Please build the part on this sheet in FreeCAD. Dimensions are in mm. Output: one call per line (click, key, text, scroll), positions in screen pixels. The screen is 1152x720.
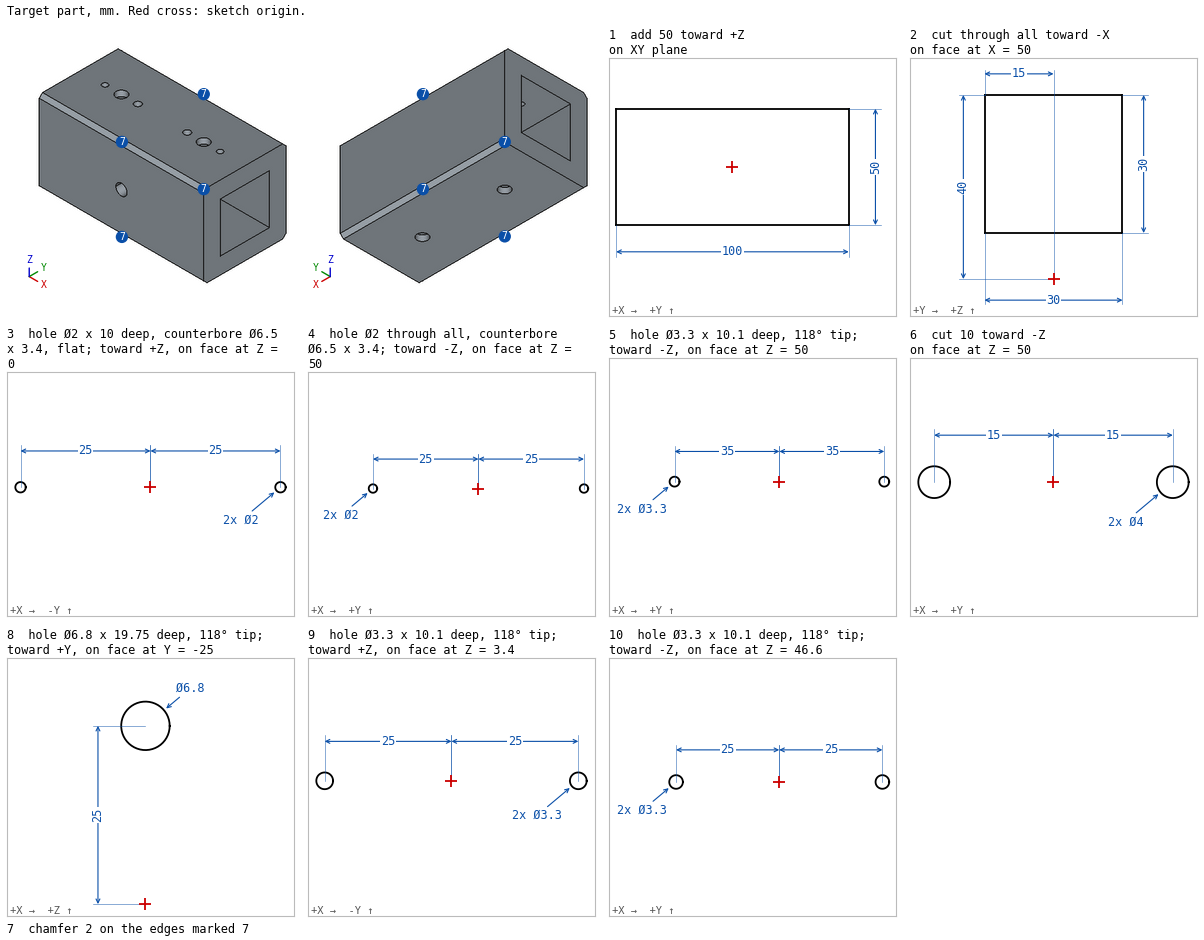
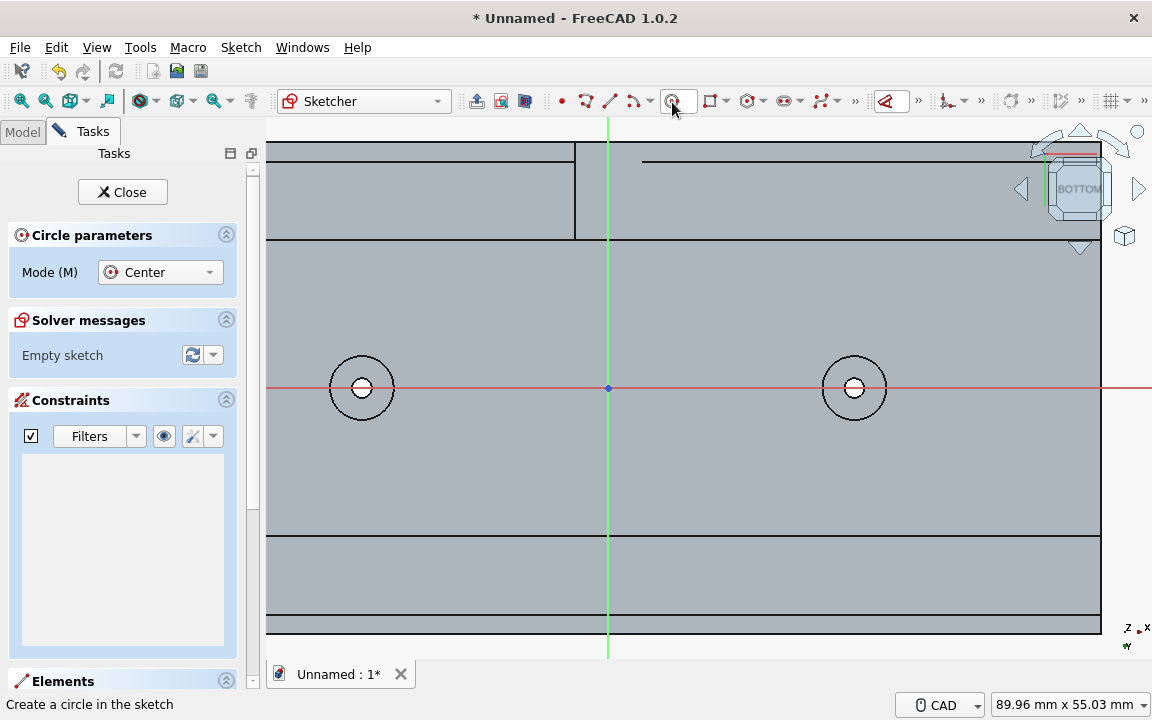
scroll(854, 388, up, 2)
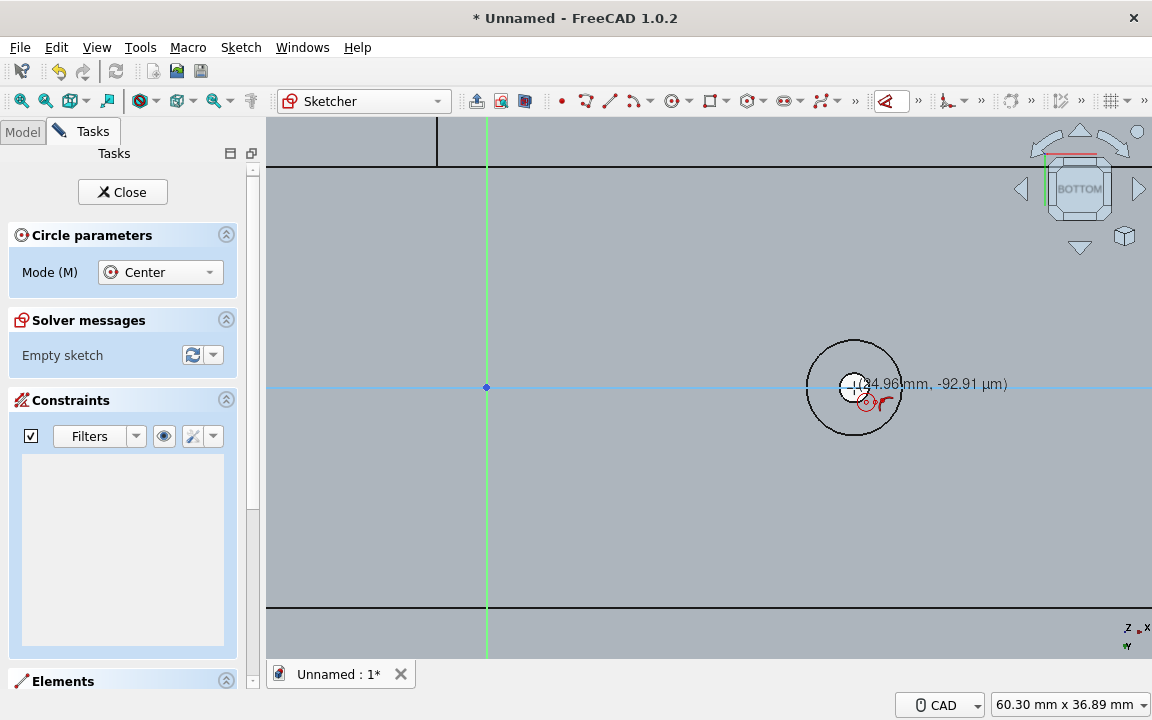
click(854, 388)
move(871, 371)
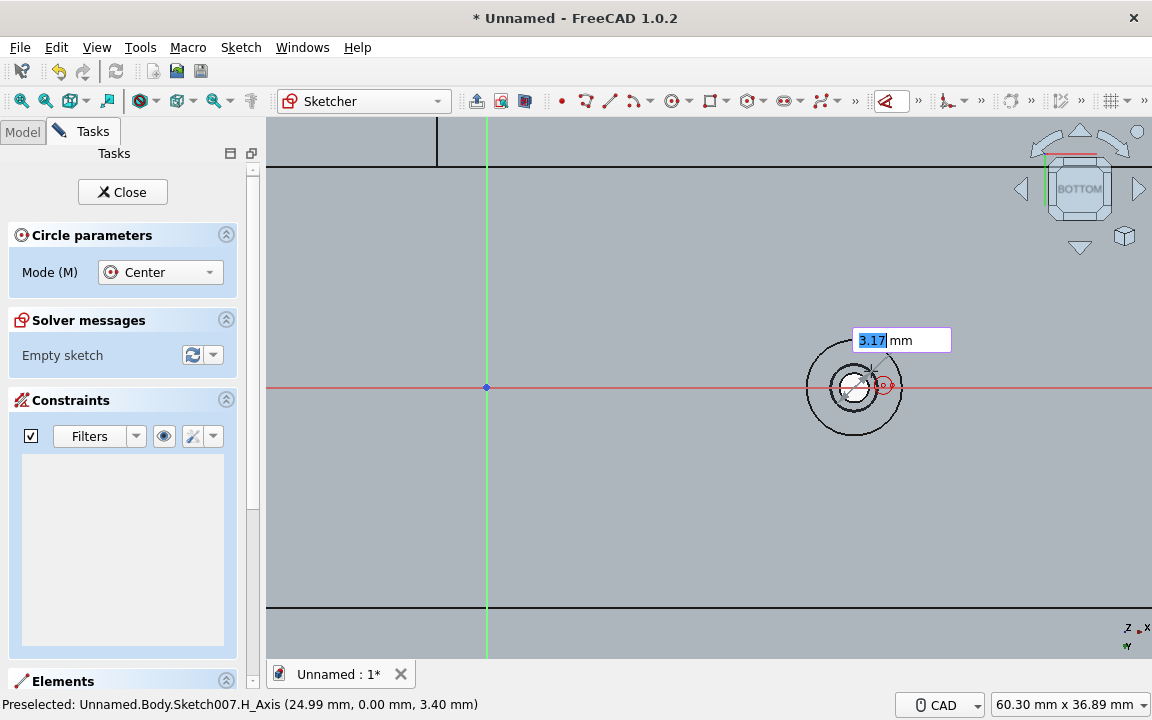
text(3.3)
key(Return)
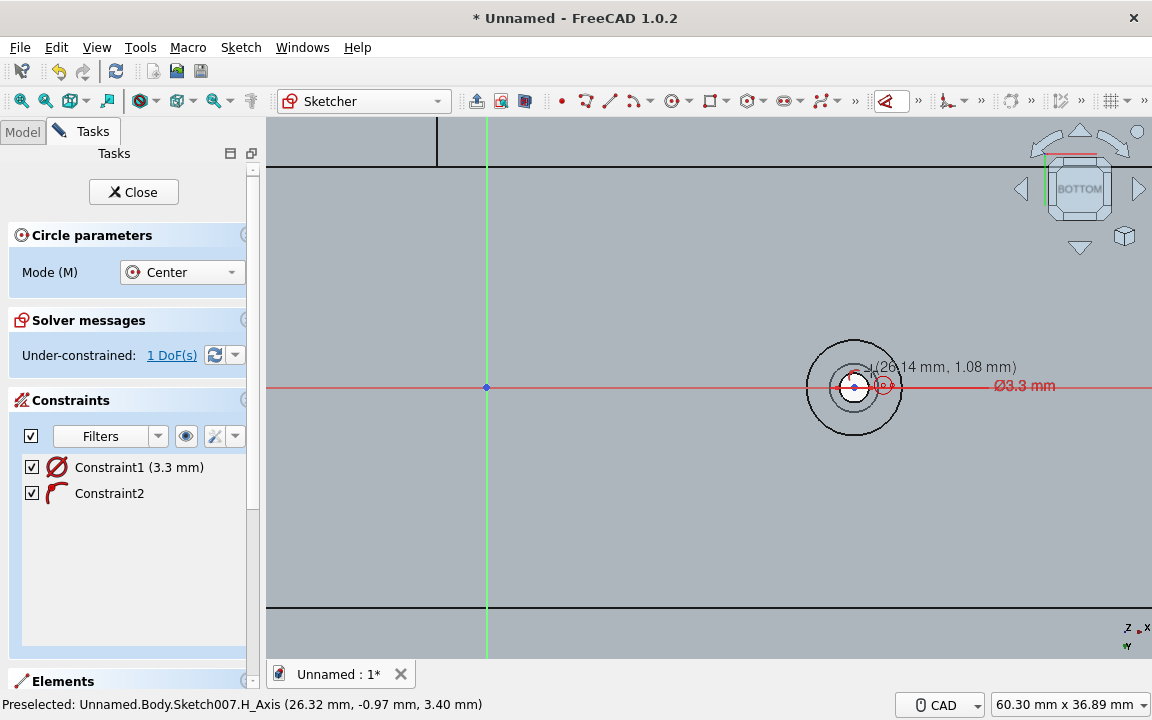
scroll(953, 388, down, 2)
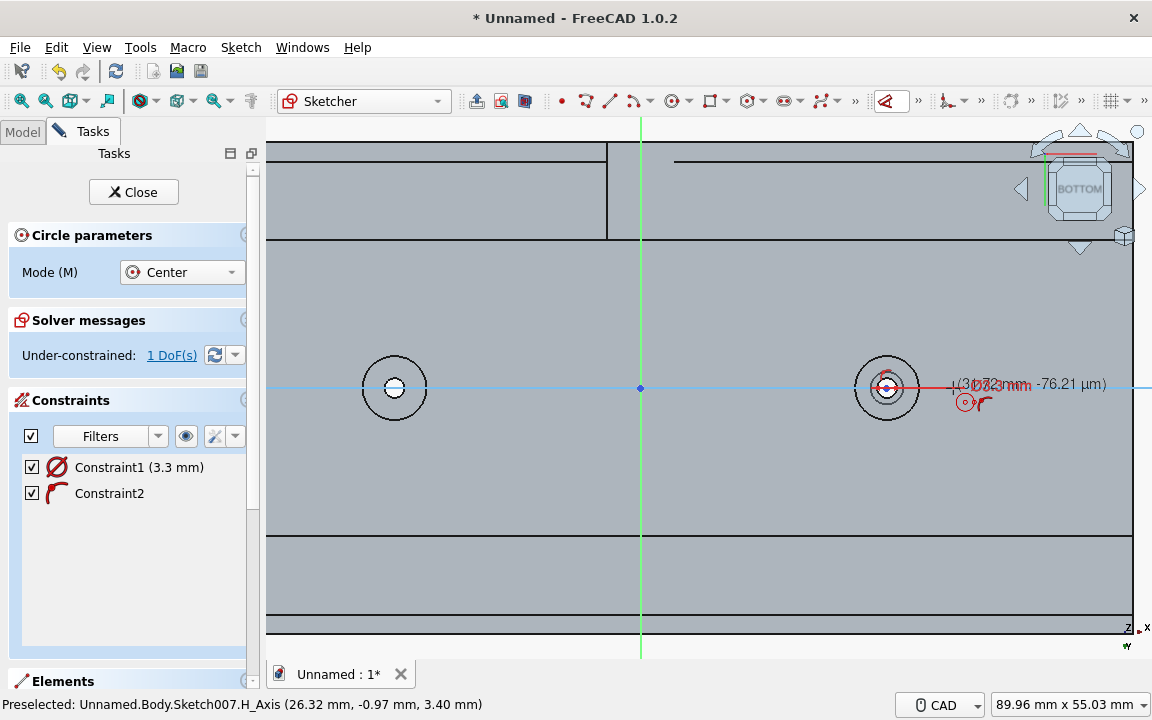
scroll(395, 388, up, 2)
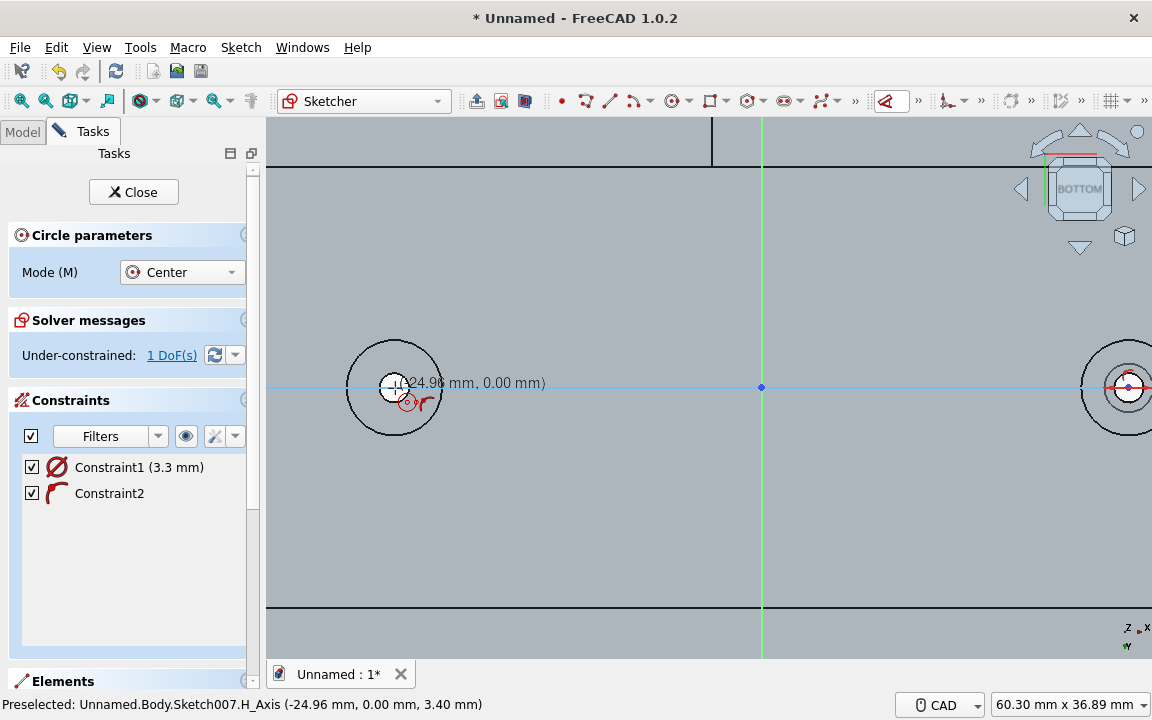
click(394, 388)
move(411, 371)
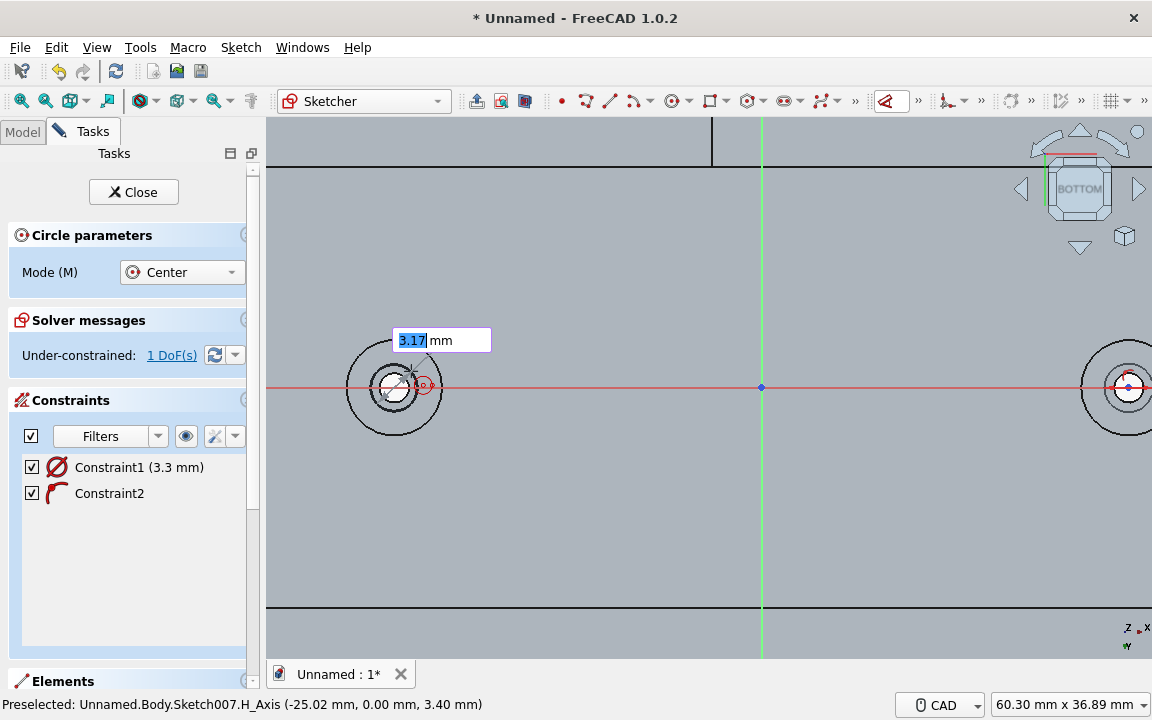
text(3.3)
key(Return)
key(Escape)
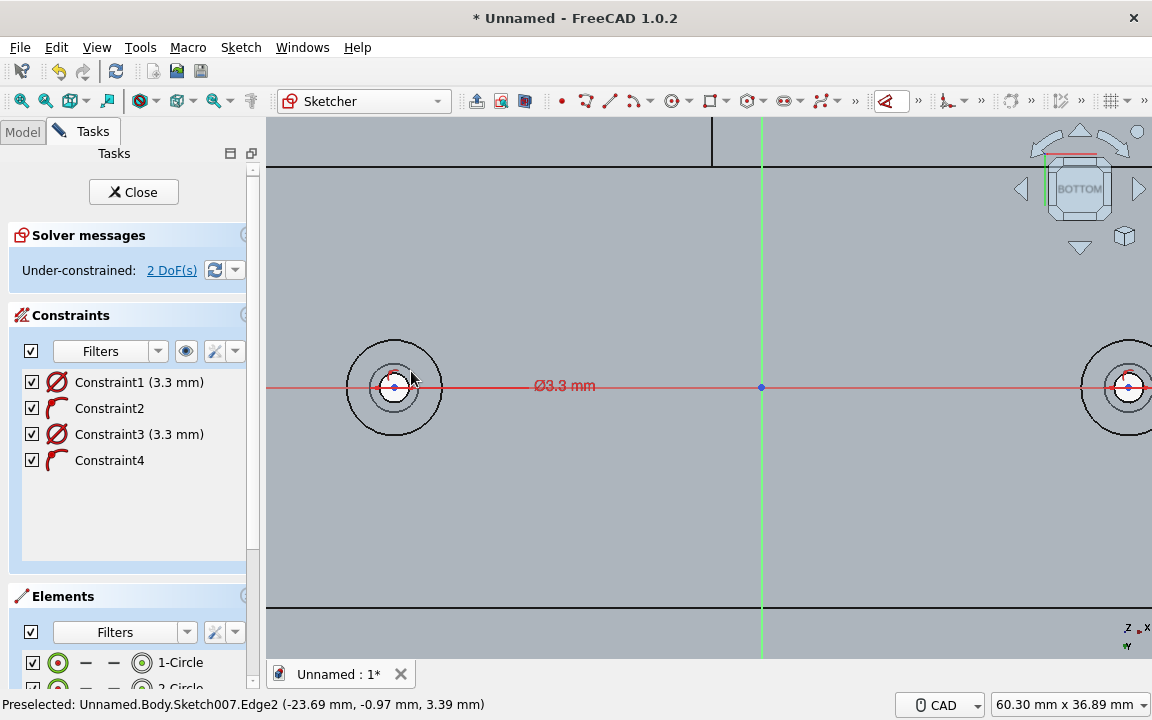
scroll(394, 388, down, 2)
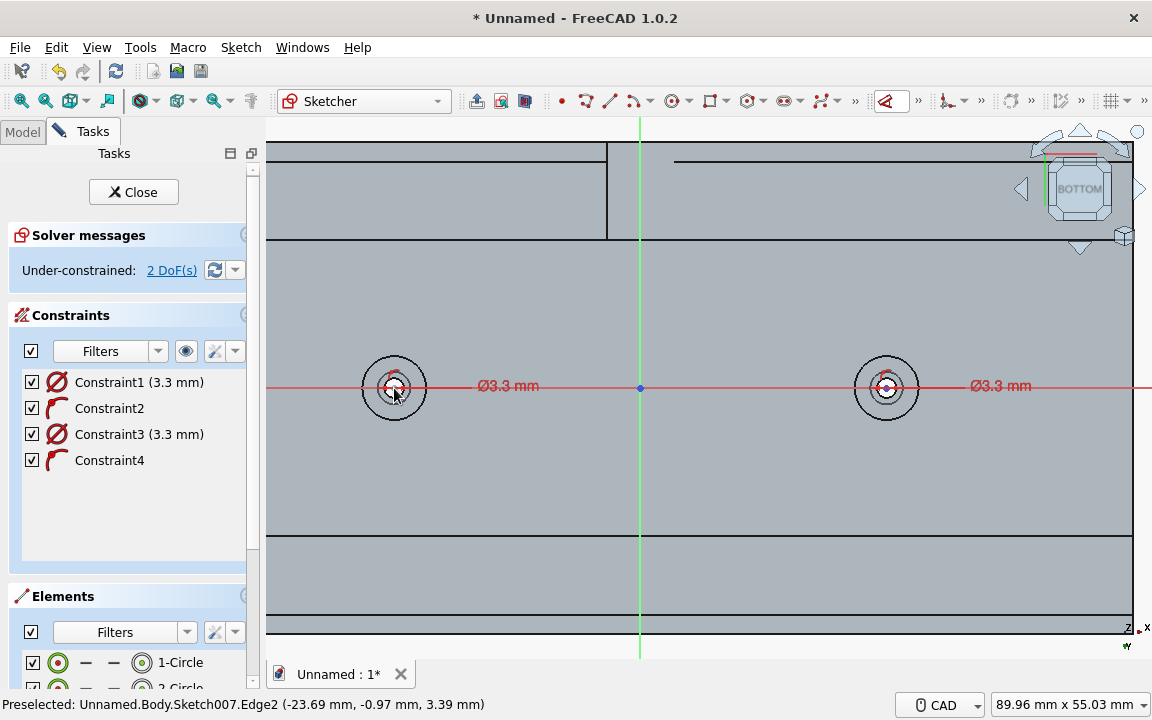
click(887, 388)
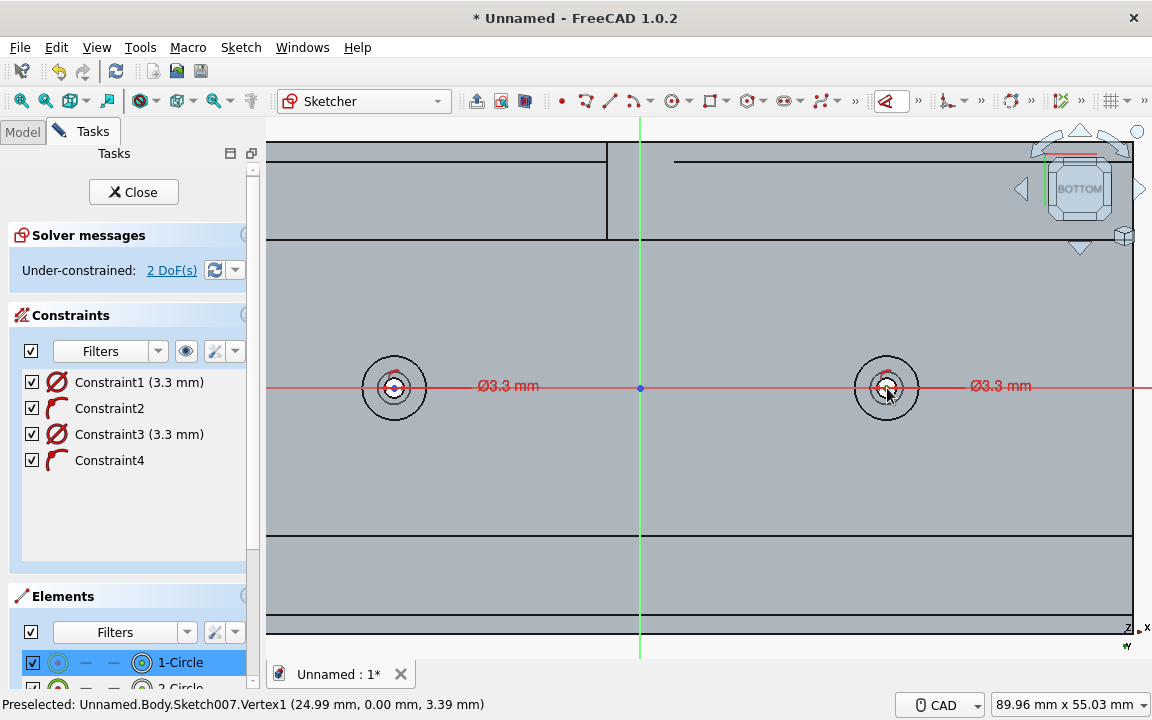
click(904, 102)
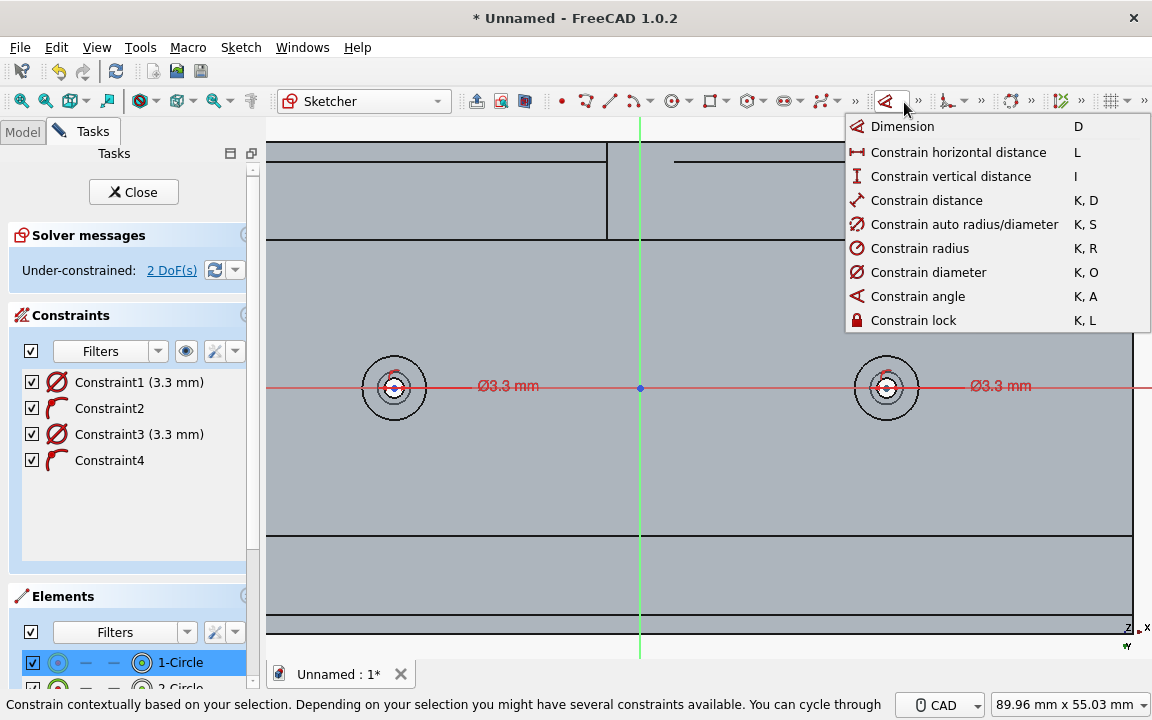
click(998, 152)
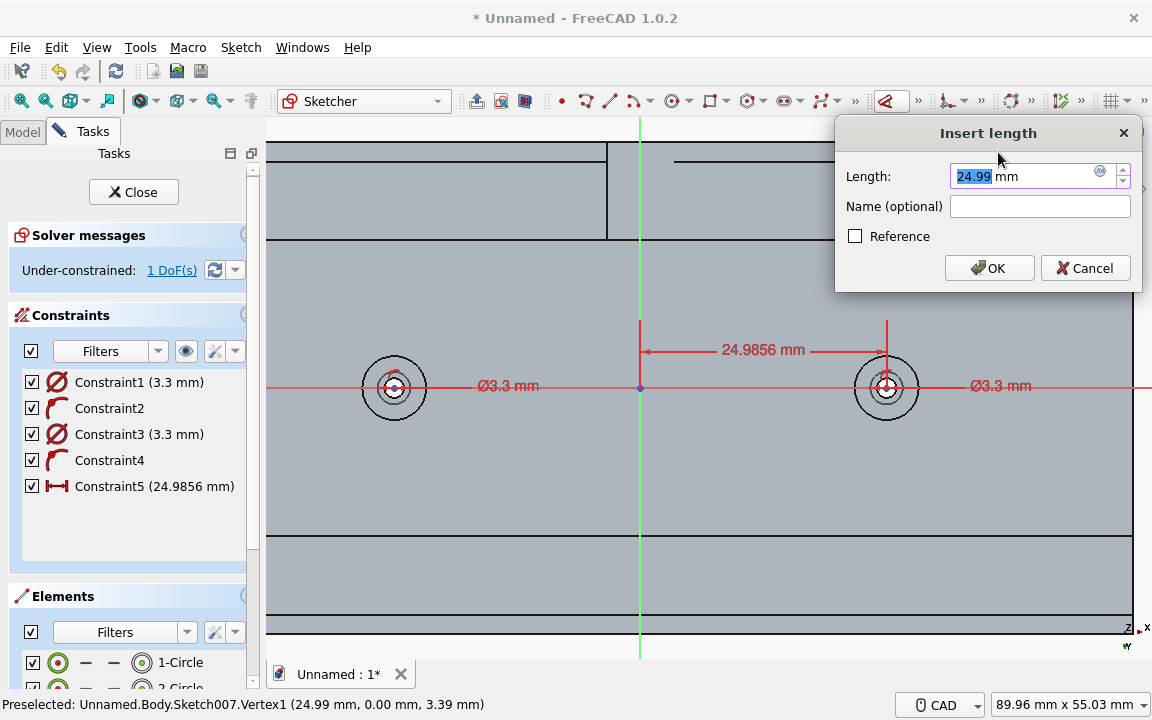
text(25)
key(Return)